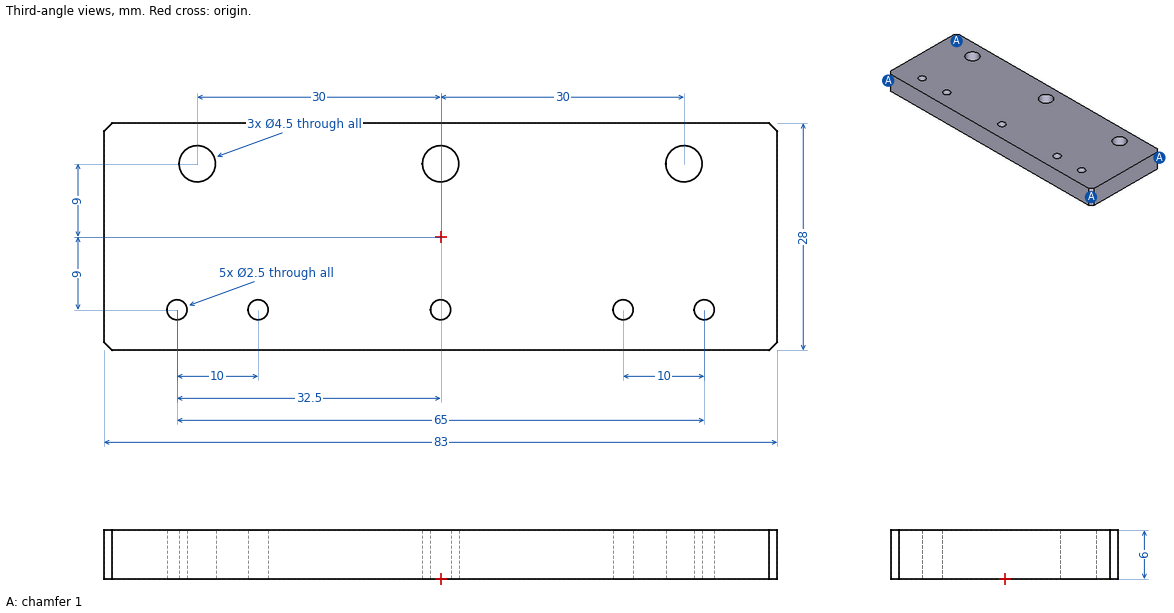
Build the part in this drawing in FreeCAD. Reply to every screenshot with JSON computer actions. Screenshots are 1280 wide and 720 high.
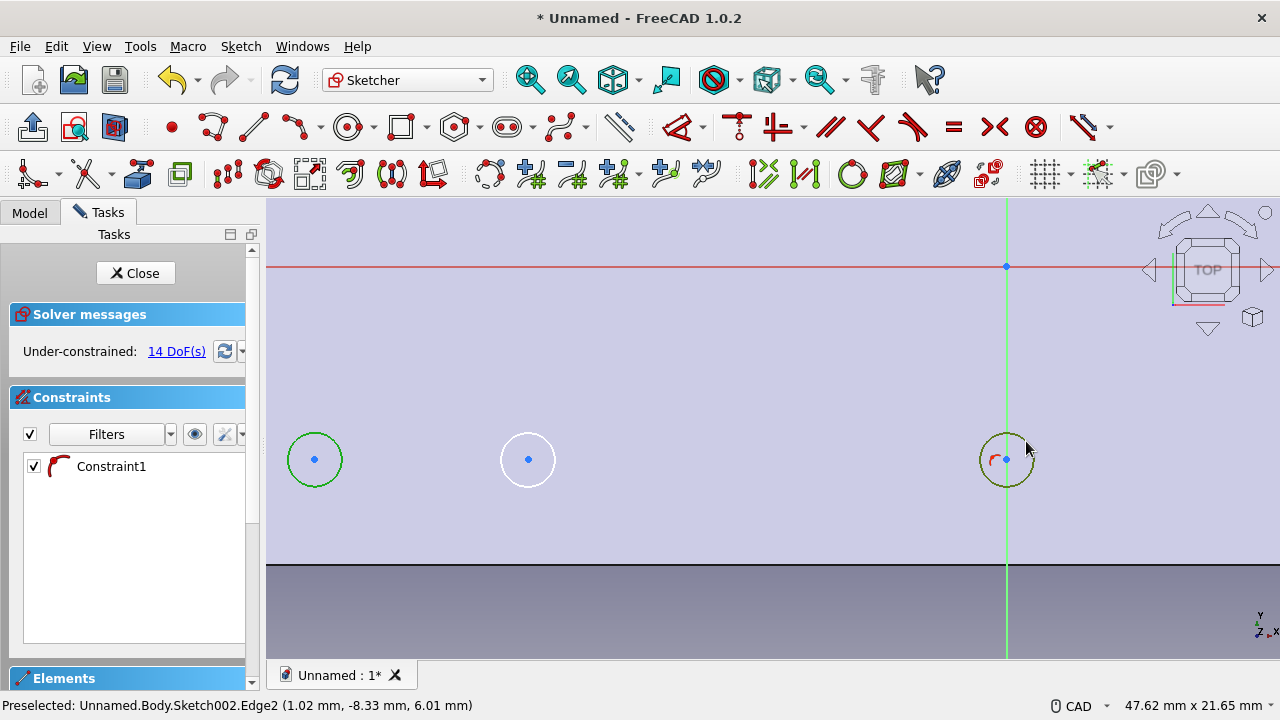
{"action": "scroll", "coordinate": [529, 459], "scroll_direction": "down", "scroll_amount": 5}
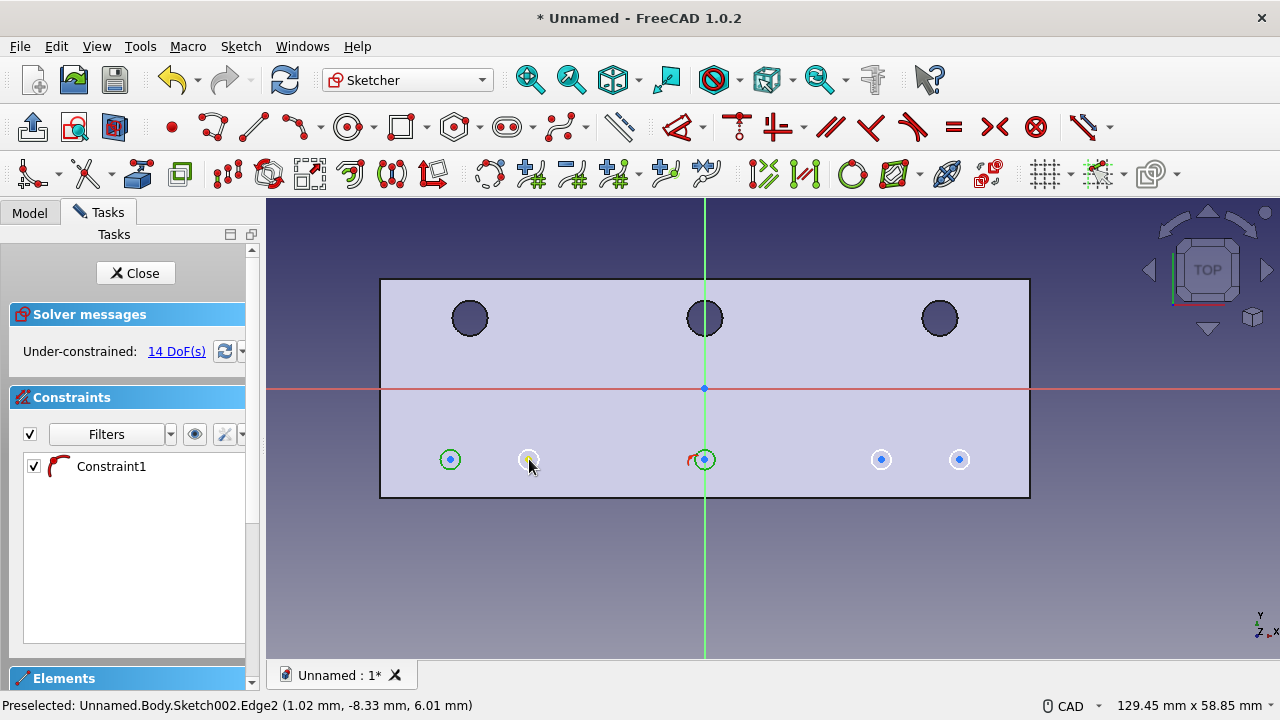
{"action": "scroll", "coordinate": [966, 453], "scroll_direction": "up", "scroll_amount": 2}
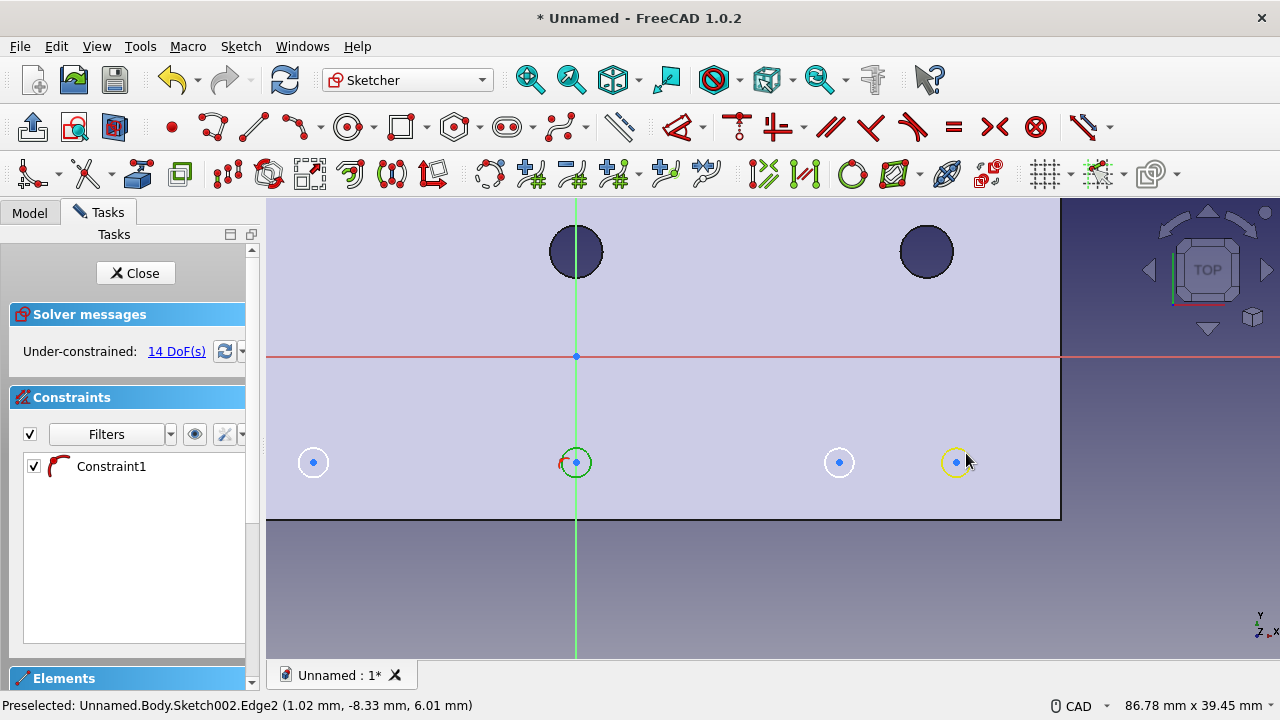
{"action": "left_click", "coordinate": [966, 453]}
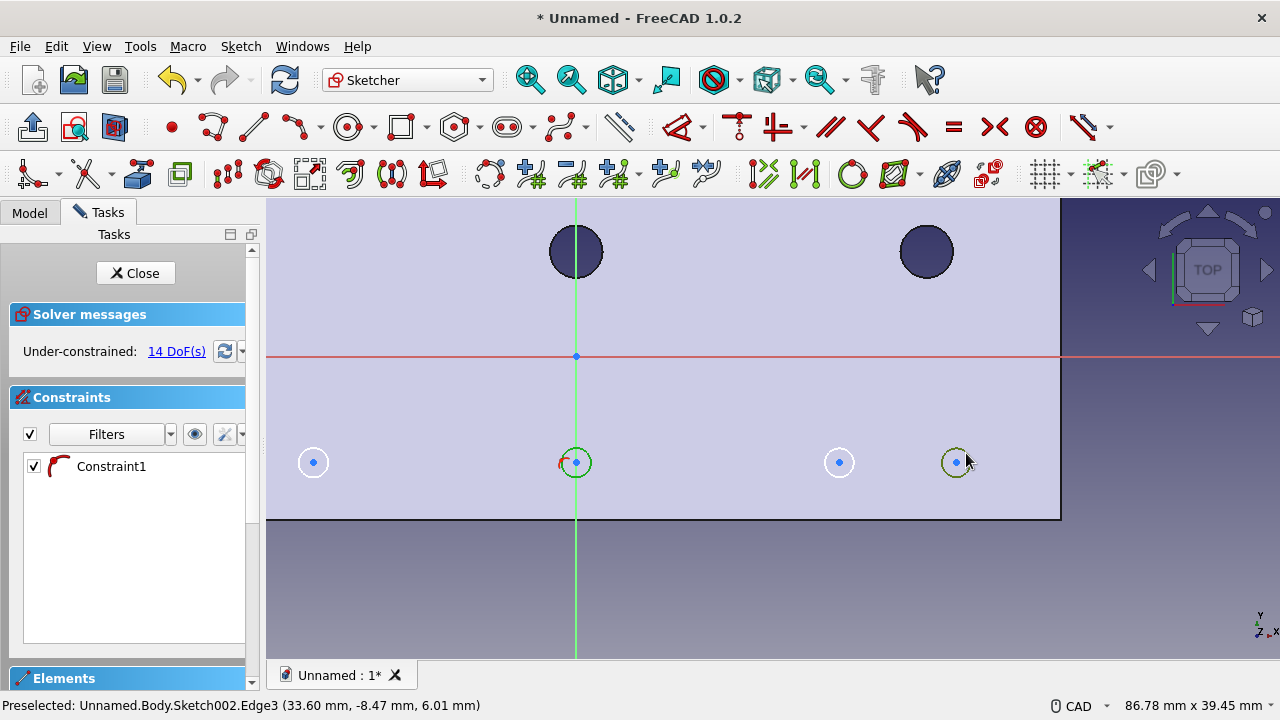
{"action": "left_click", "coordinate": [849, 453]}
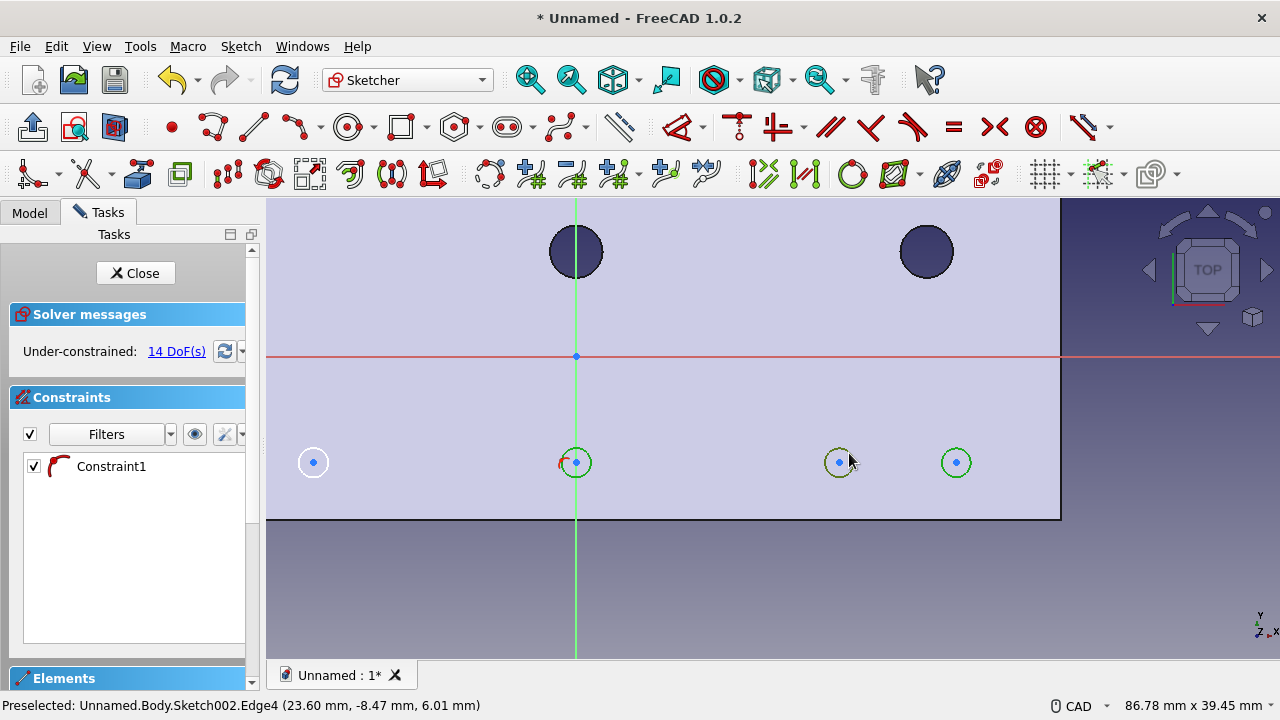
{"action": "left_click", "coordinate": [324, 452]}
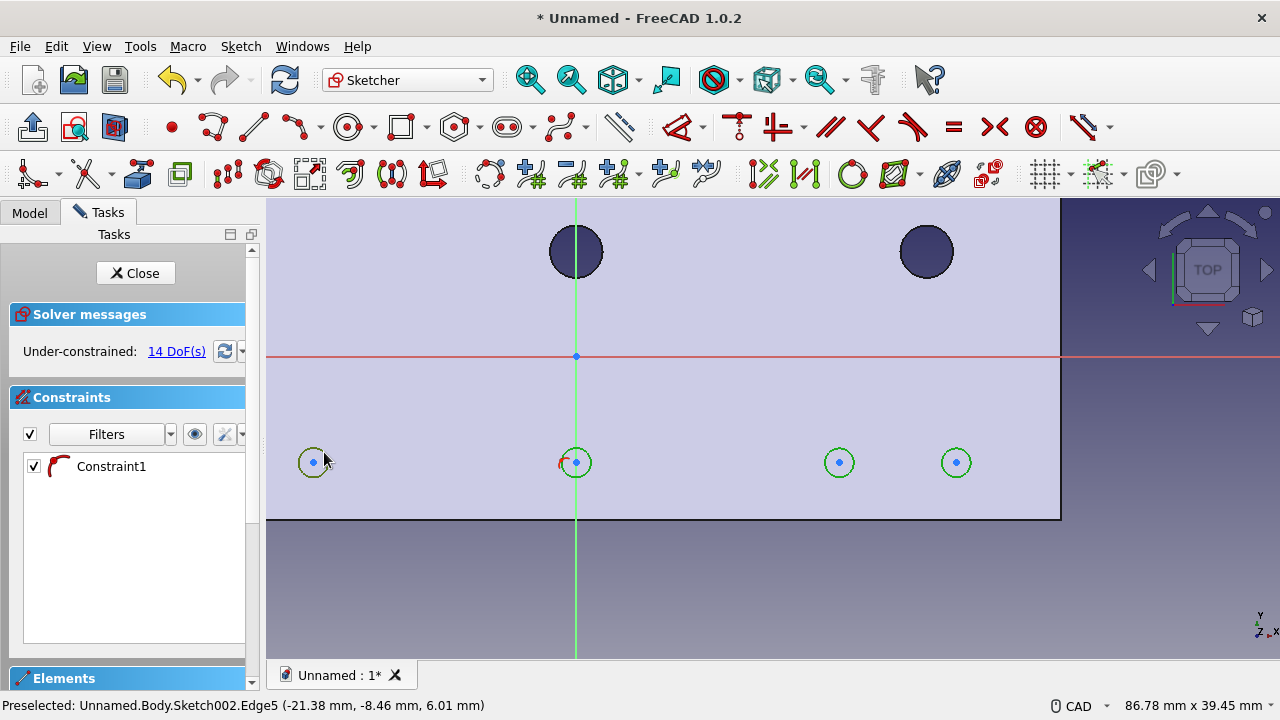
{"action": "left_click", "coordinate": [954, 128]}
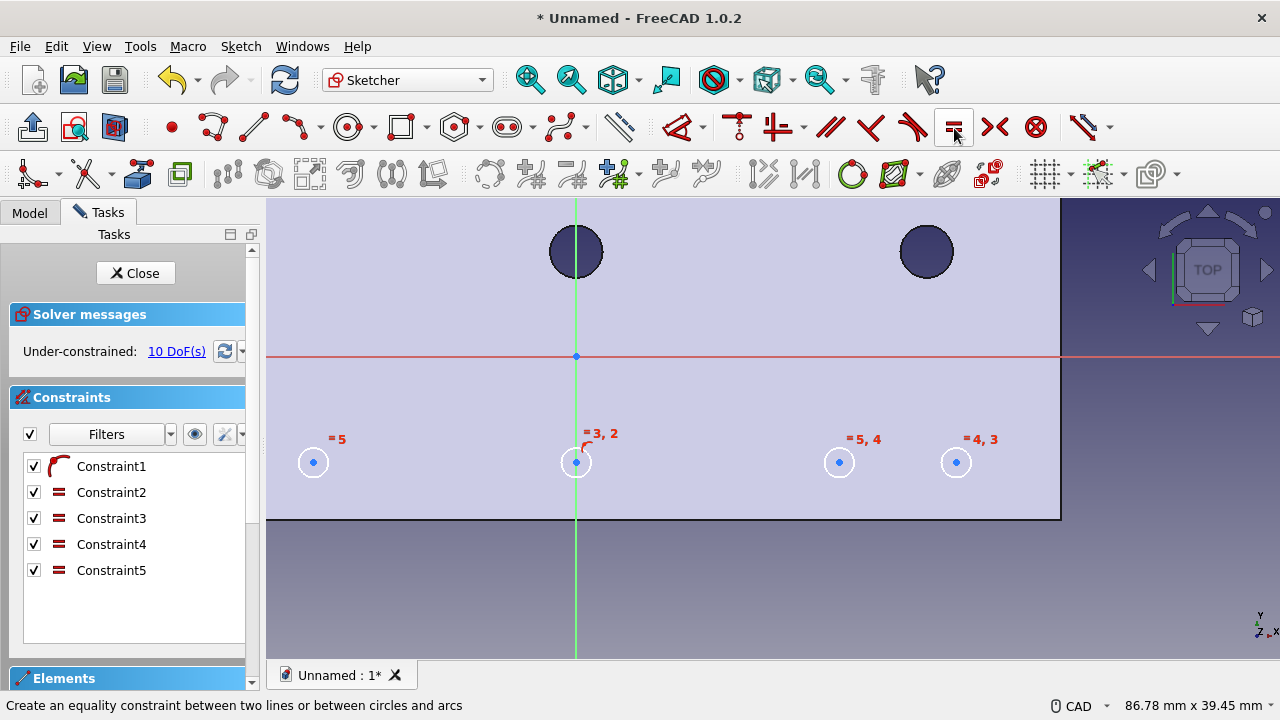
{"action": "key", "text": "d"}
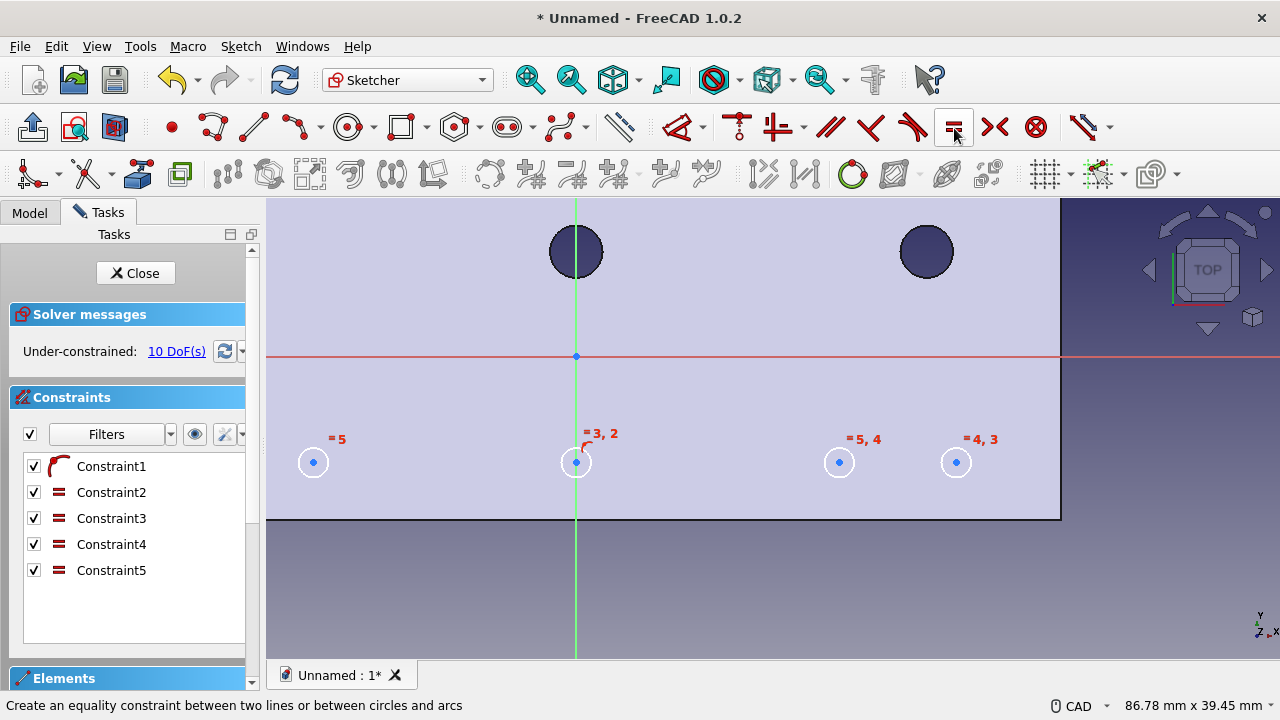
{"action": "scroll", "coordinate": [965, 452], "scroll_direction": "down", "scroll_amount": 2}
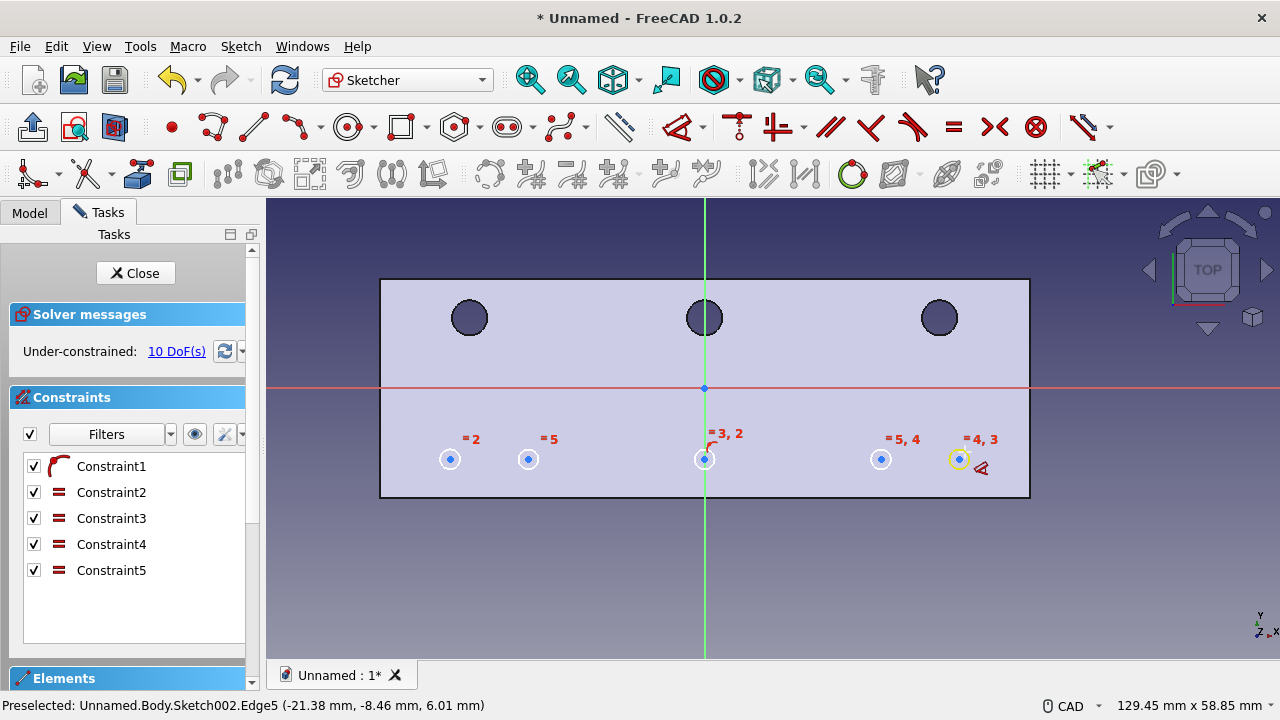
{"action": "scroll", "coordinate": [457, 452], "scroll_direction": "up", "scroll_amount": 4}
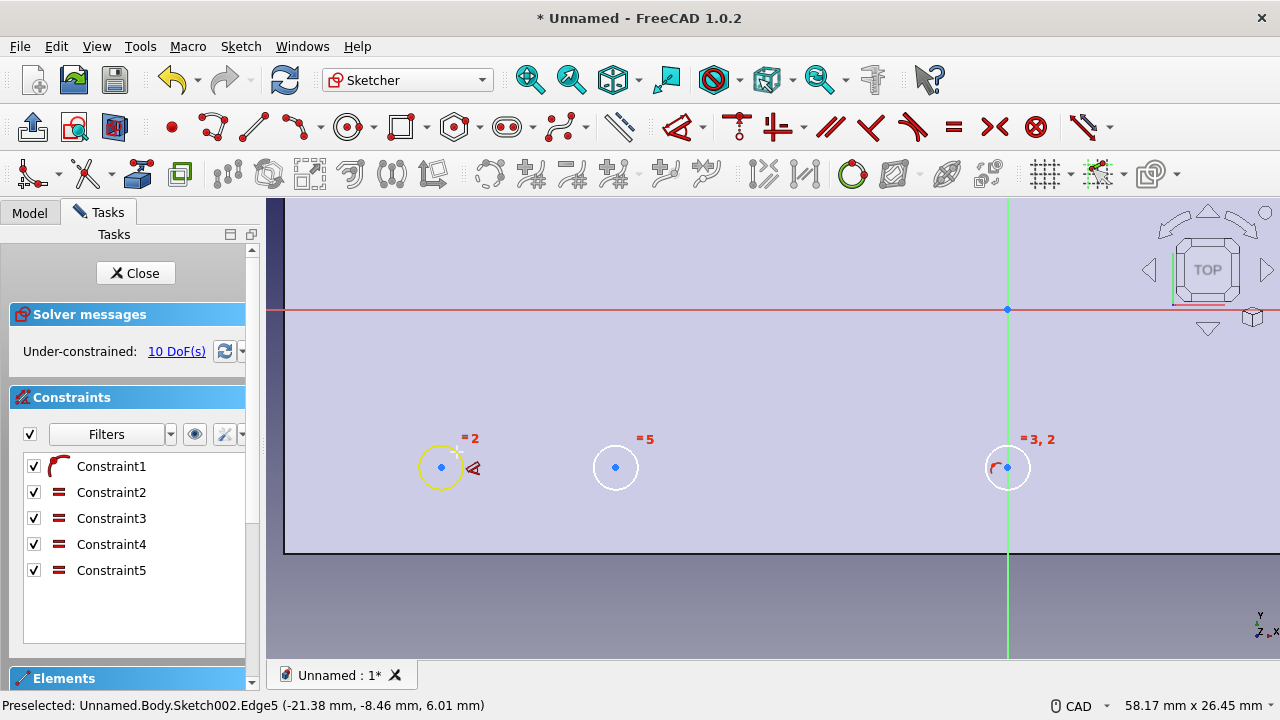
{"action": "left_click", "coordinate": [457, 452]}
{"action": "left_click", "coordinate": [480, 429]}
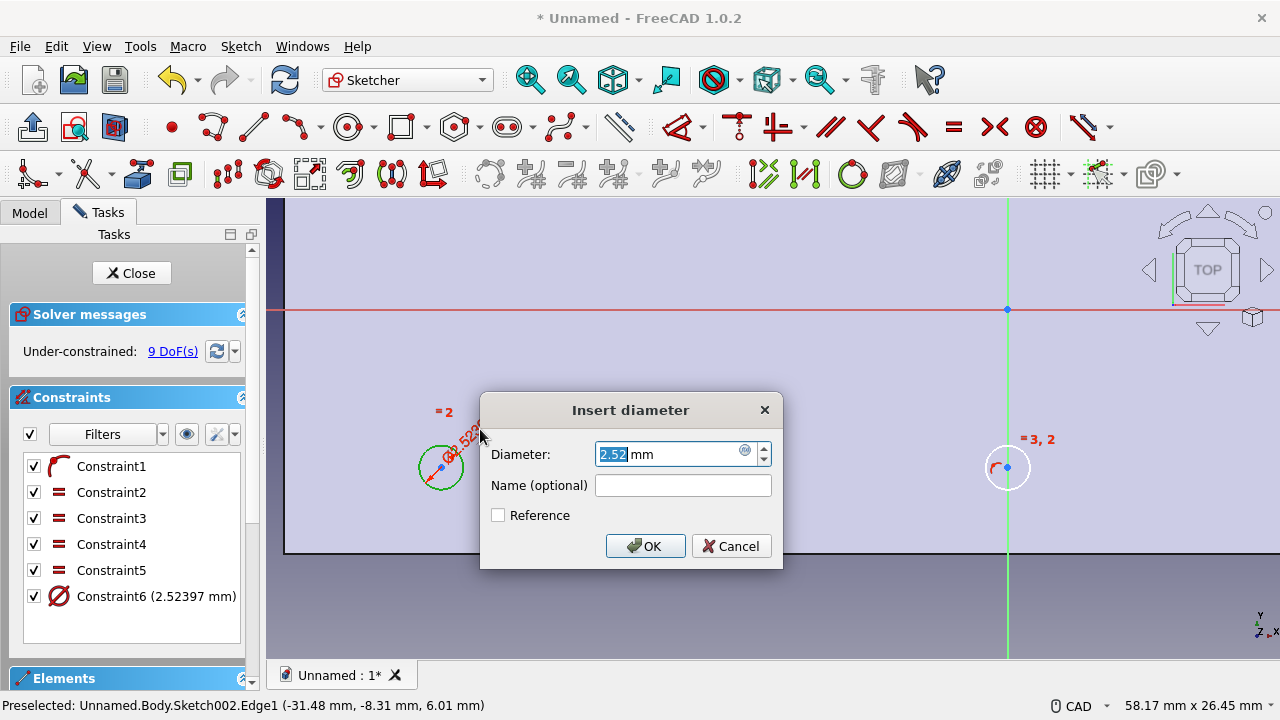
{"action": "type", "text": "2.5"}
{"action": "key", "text": "Return"}